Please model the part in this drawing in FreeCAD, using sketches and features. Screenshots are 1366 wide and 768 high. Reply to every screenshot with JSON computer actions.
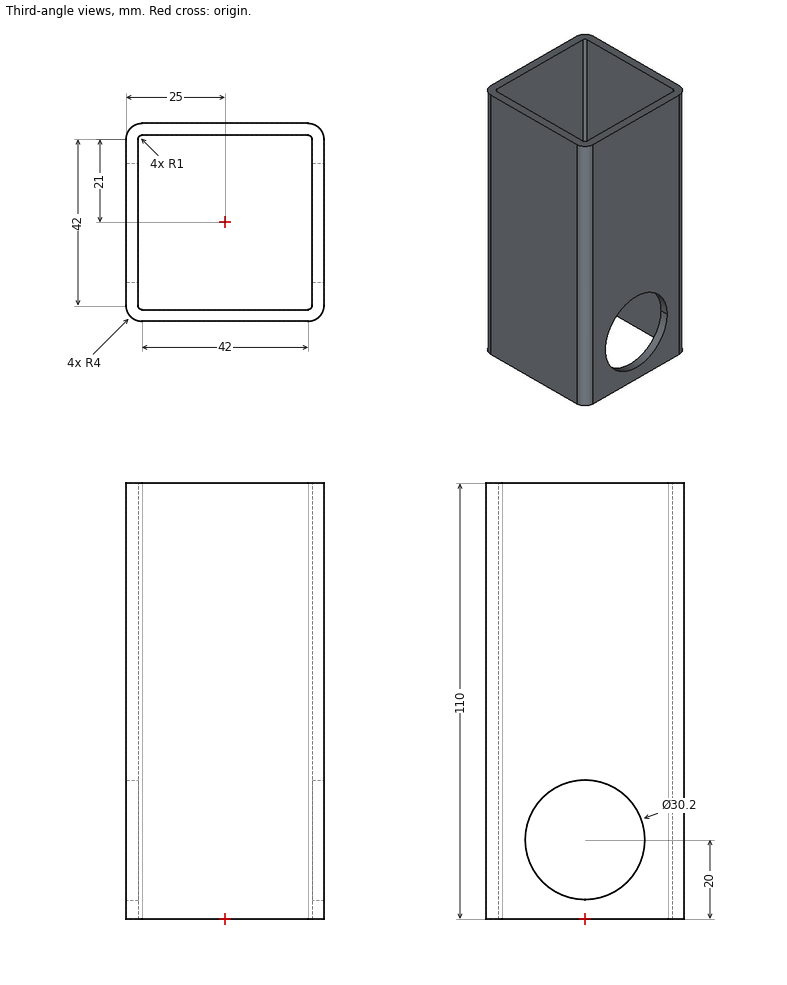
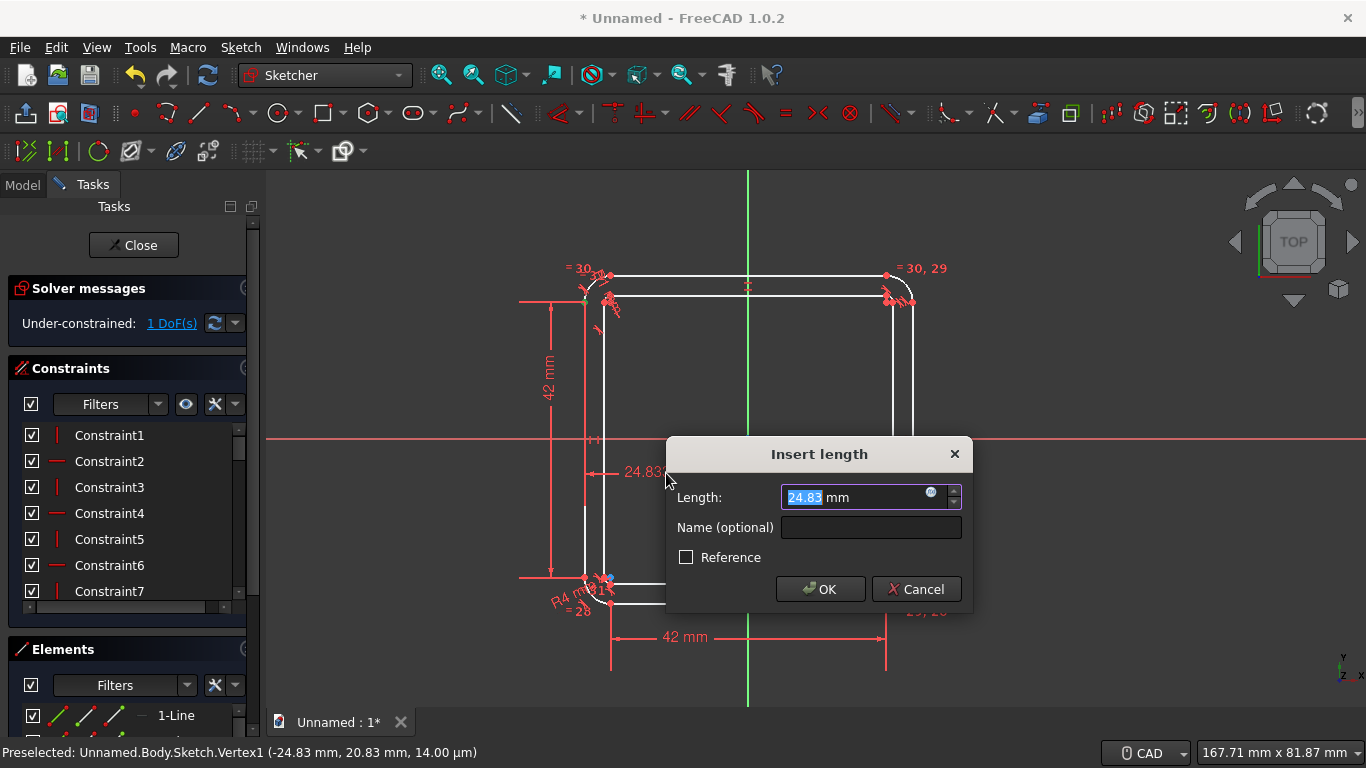
{"action": "type", "text": "25"}
{"action": "key", "text": "Return"}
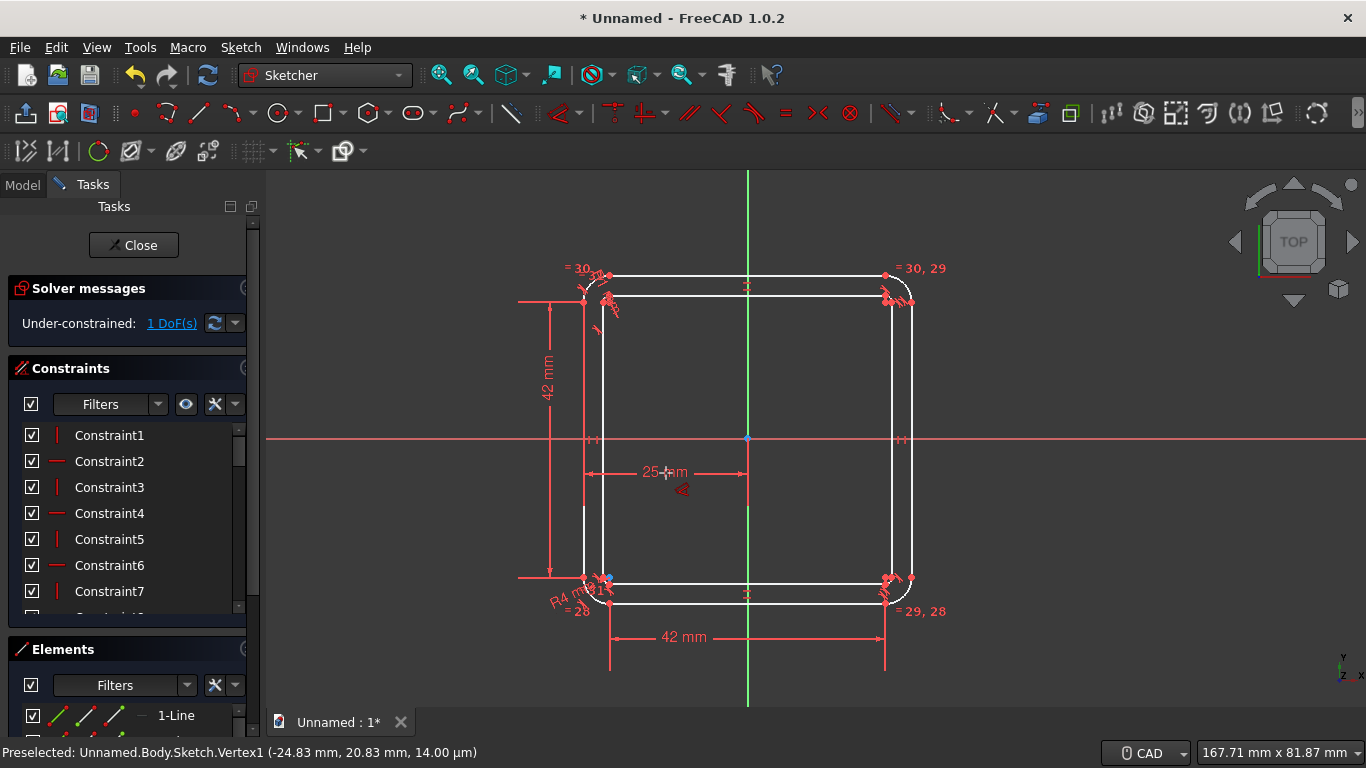
{"action": "left_click", "coordinate": [584, 302]}
{"action": "left_click", "coordinate": [550, 339]}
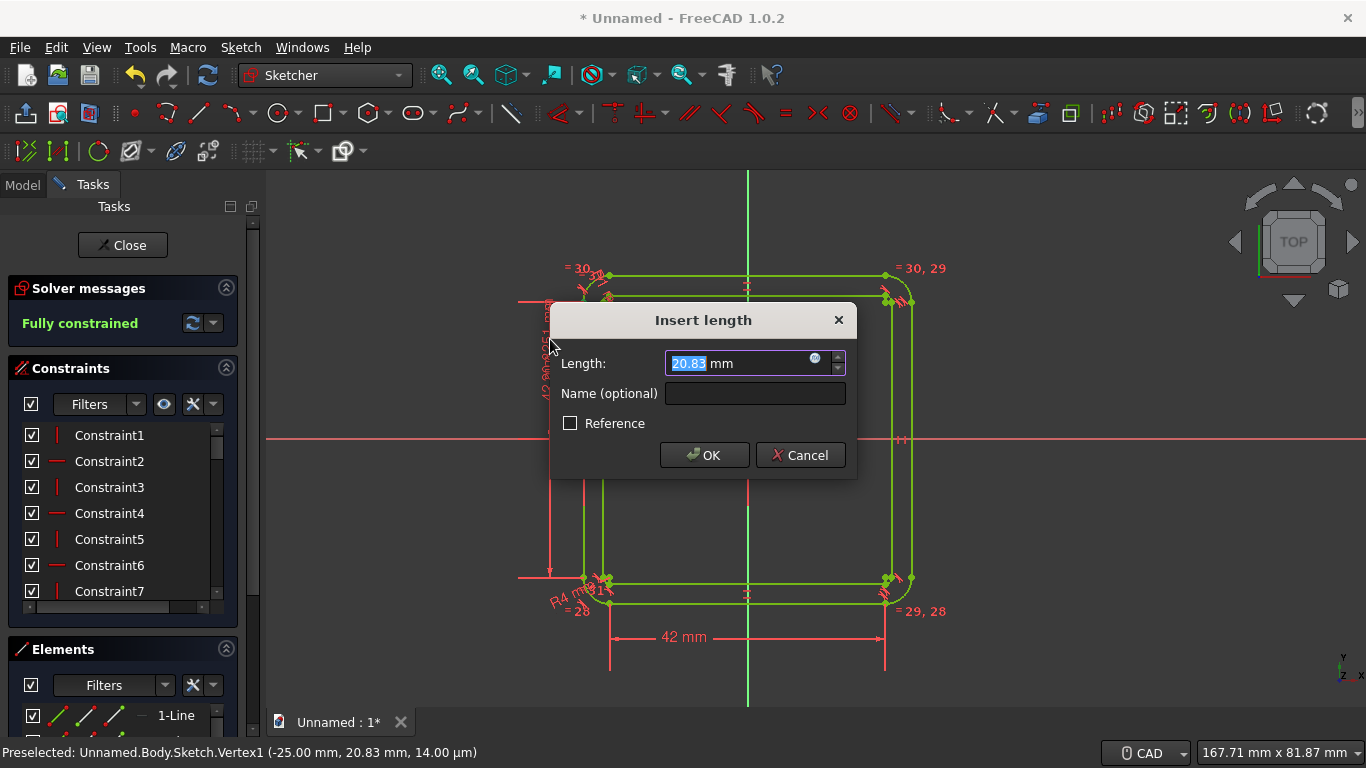
{"action": "type", "text": "21"}
{"action": "key", "text": "Return"}
{"action": "key", "text": "Escape"}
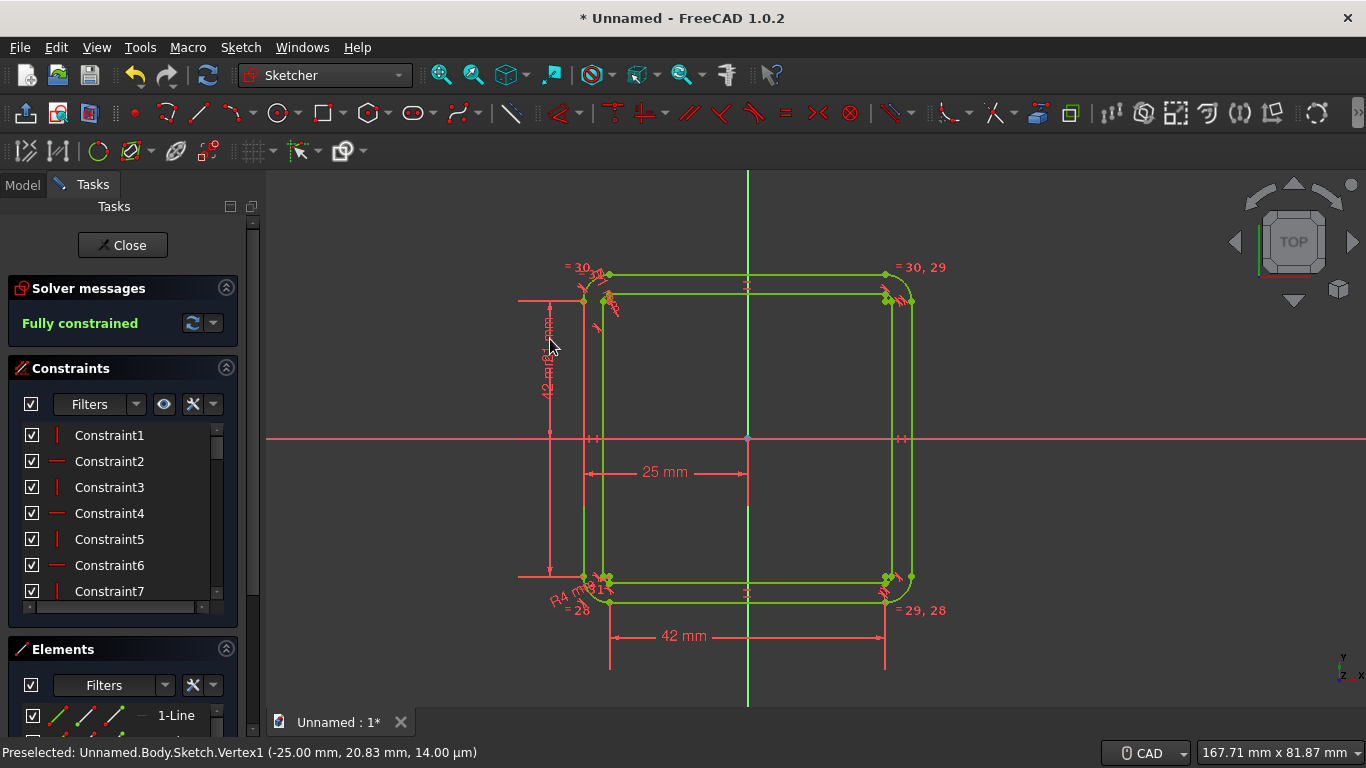
{"action": "left_click", "coordinate": [123, 245]}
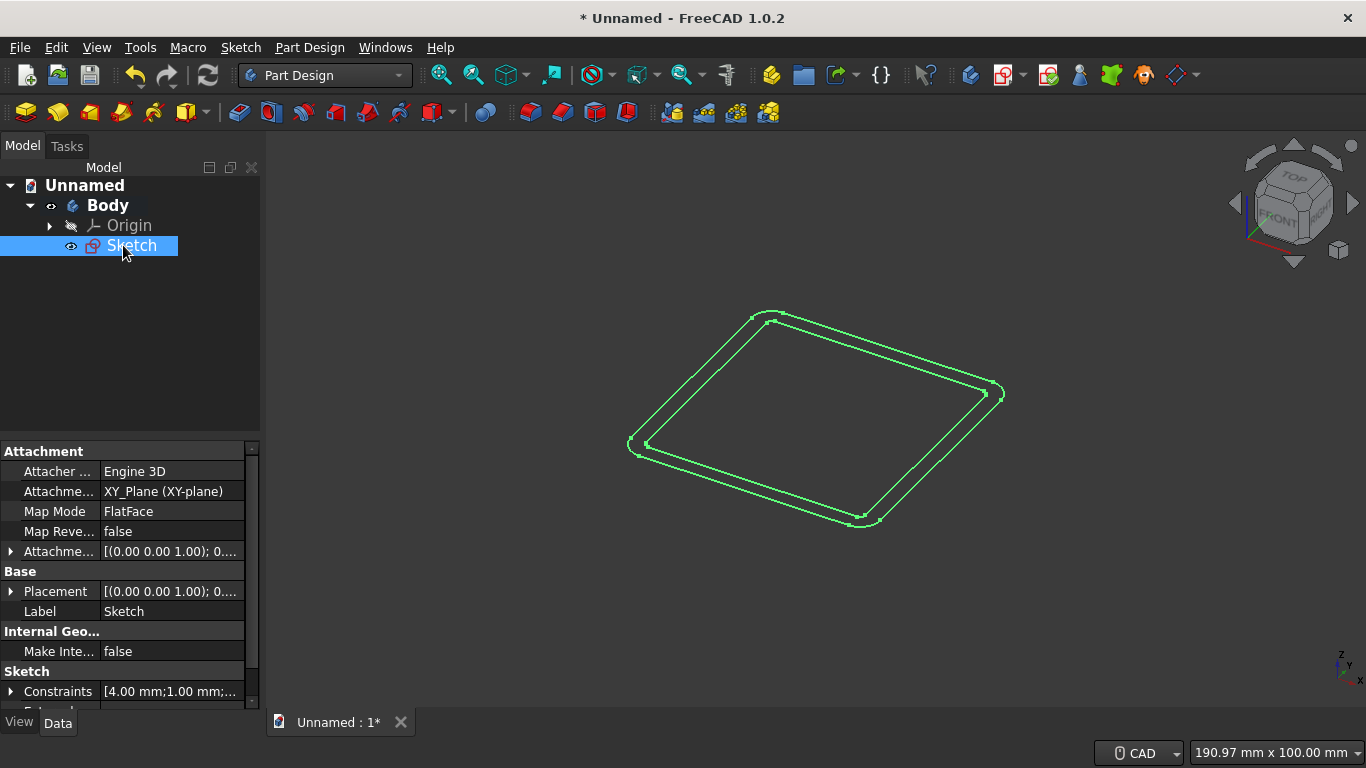
{"action": "left_click", "coordinate": [26, 112]}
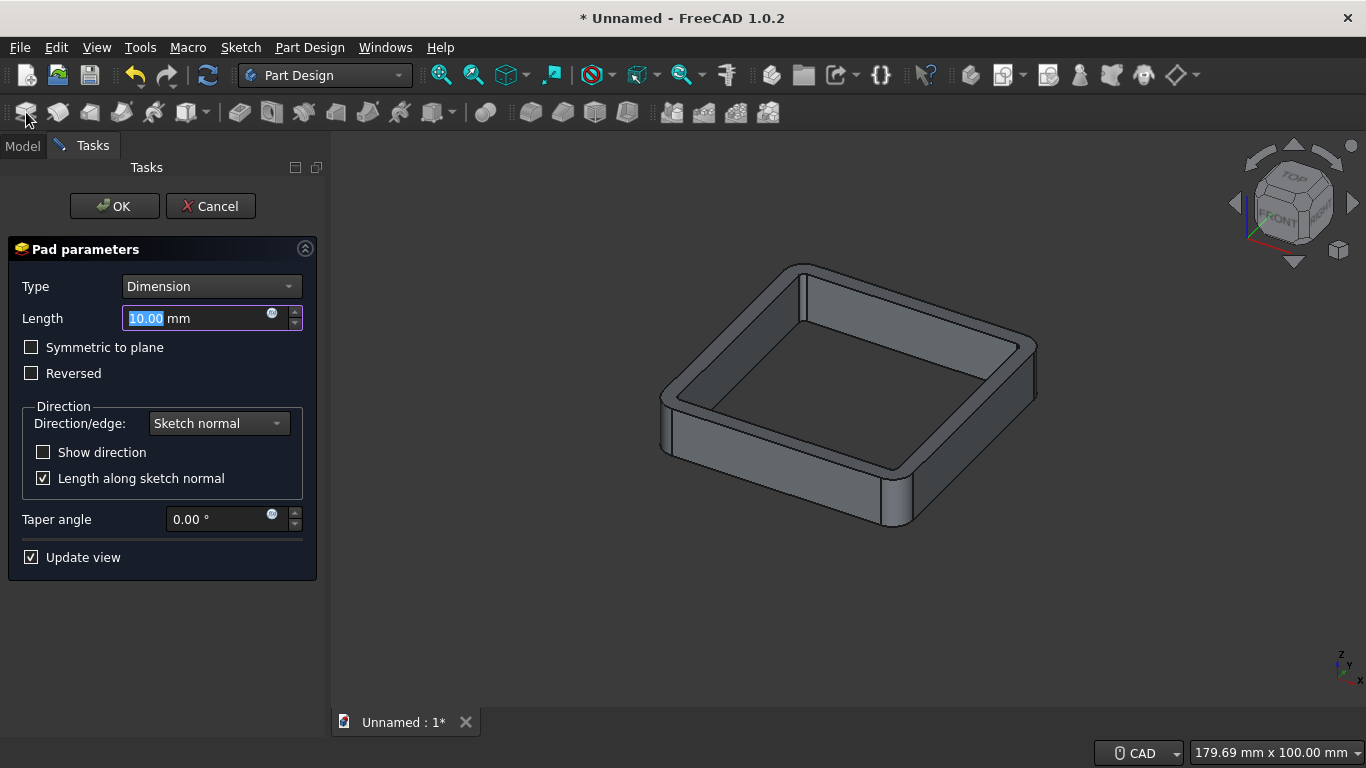
{"action": "type", "text": "110"}
{"action": "key", "text": "Tab"}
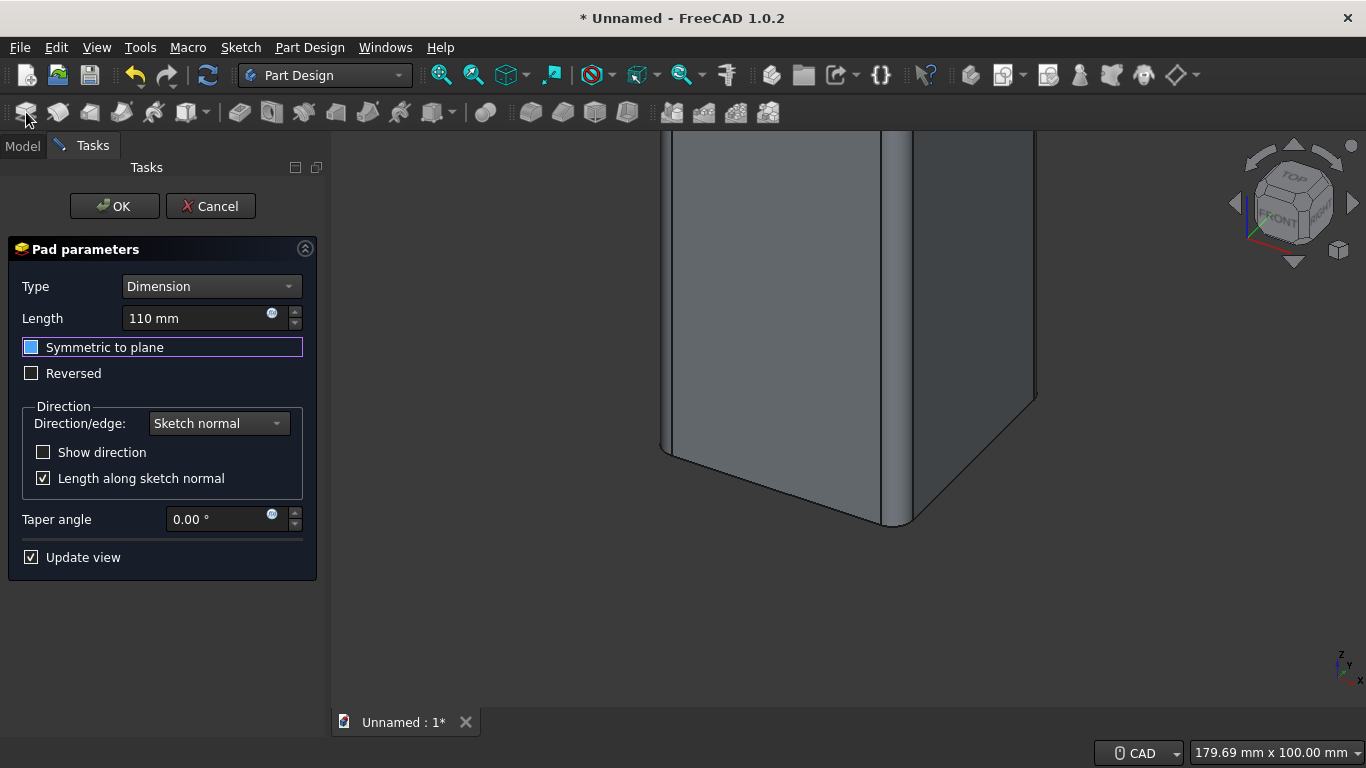
{"action": "left_click", "coordinate": [115, 206]}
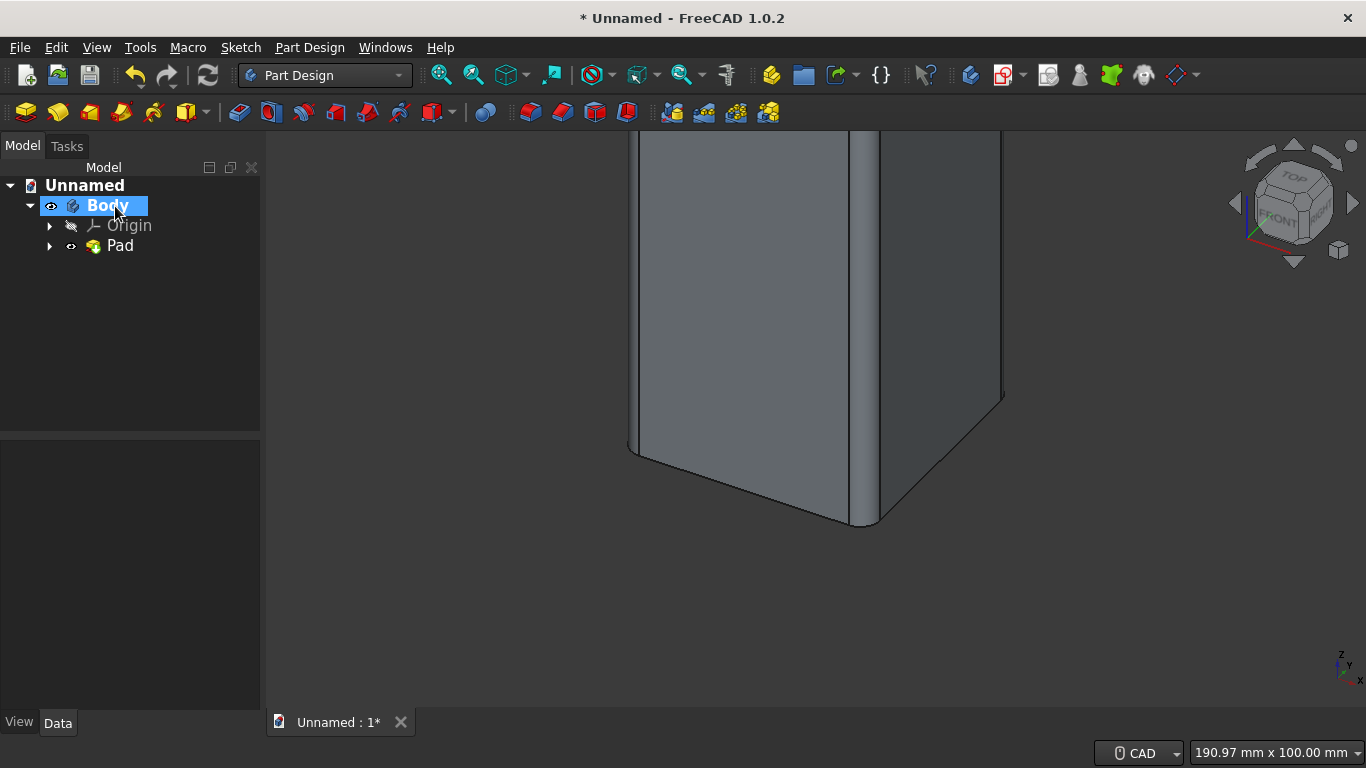
{"action": "left_click", "coordinate": [442, 76]}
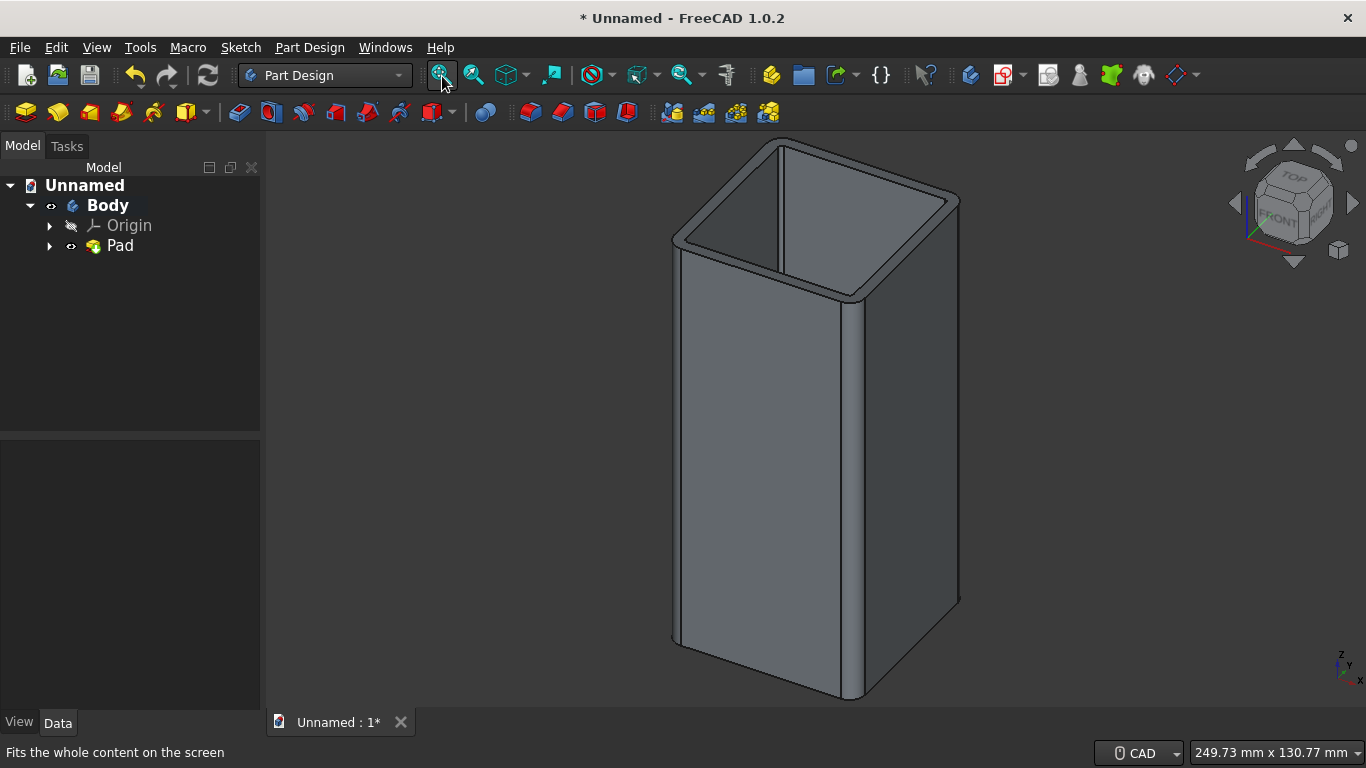
{"action": "left_click", "coordinate": [911, 336]}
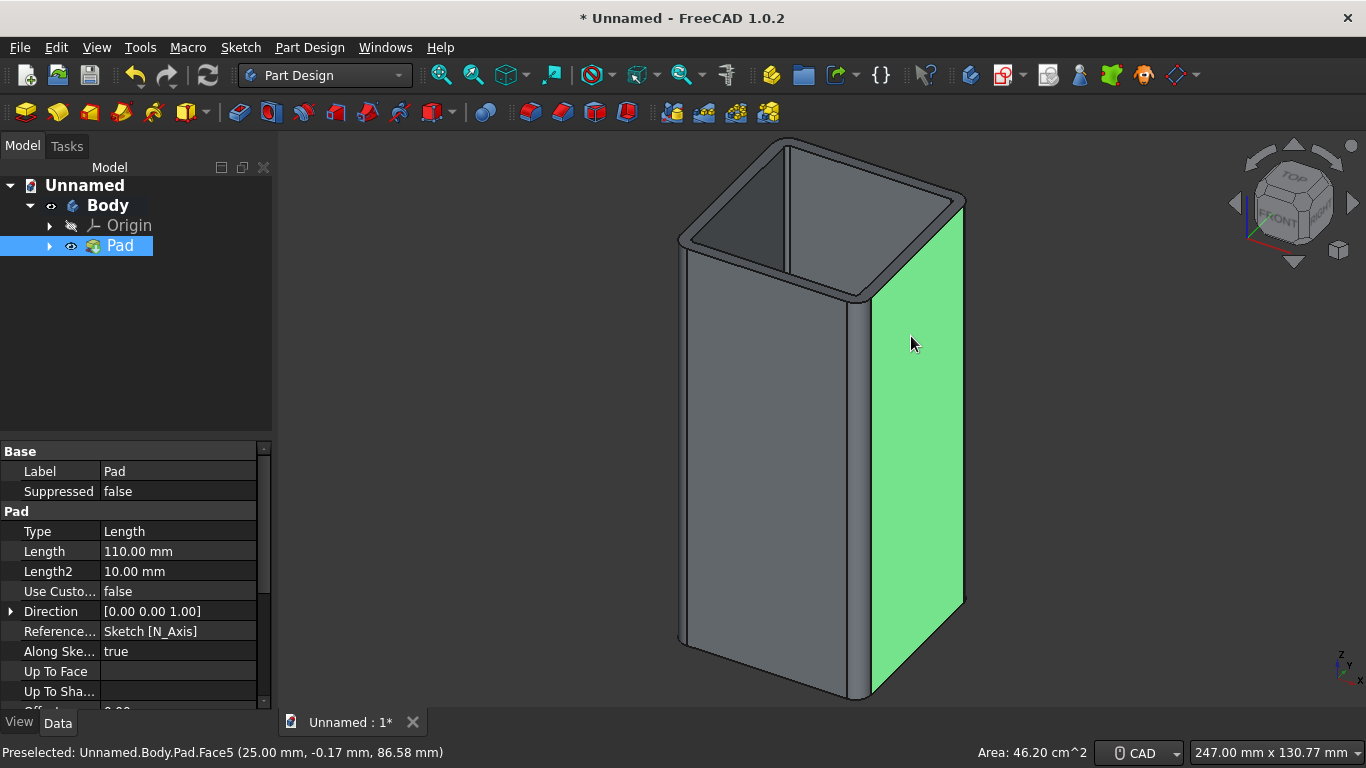
{"action": "left_click", "coordinate": [1004, 76]}